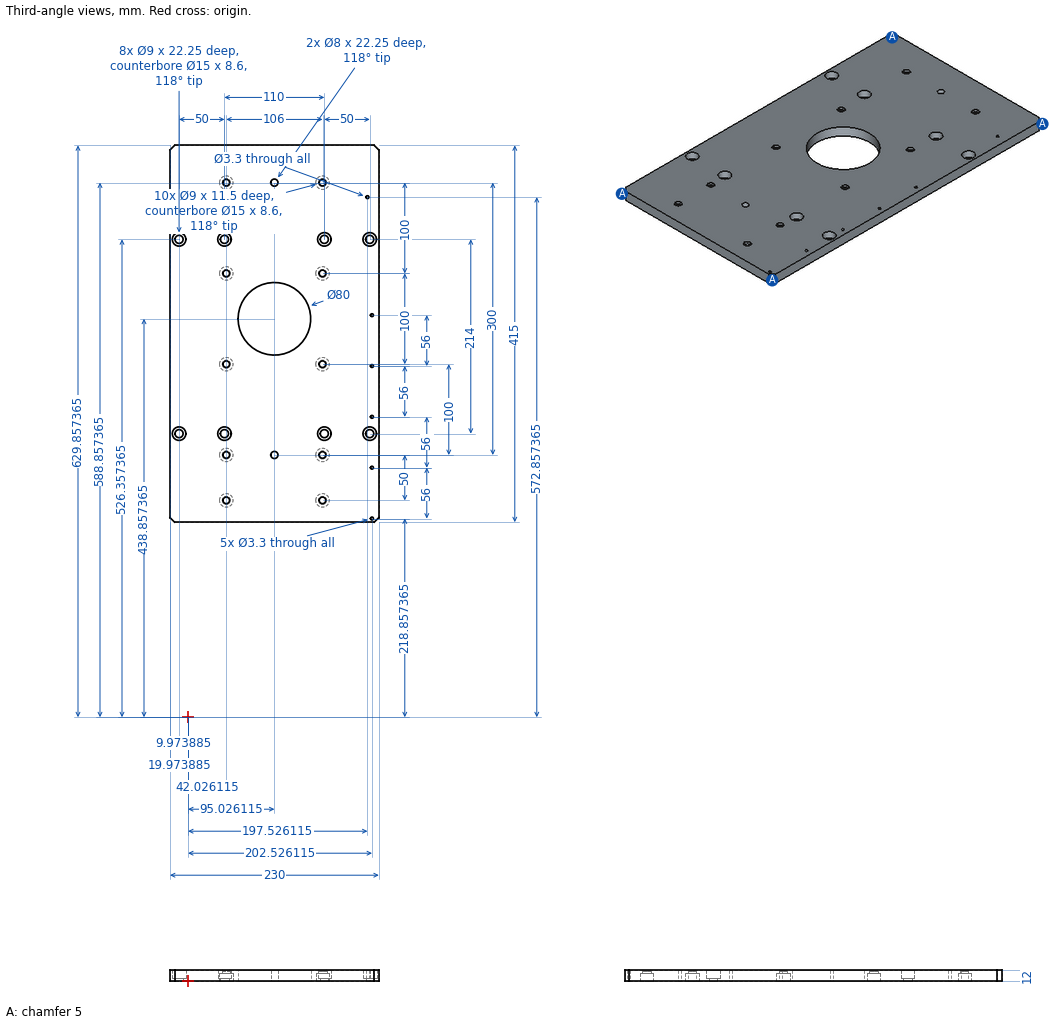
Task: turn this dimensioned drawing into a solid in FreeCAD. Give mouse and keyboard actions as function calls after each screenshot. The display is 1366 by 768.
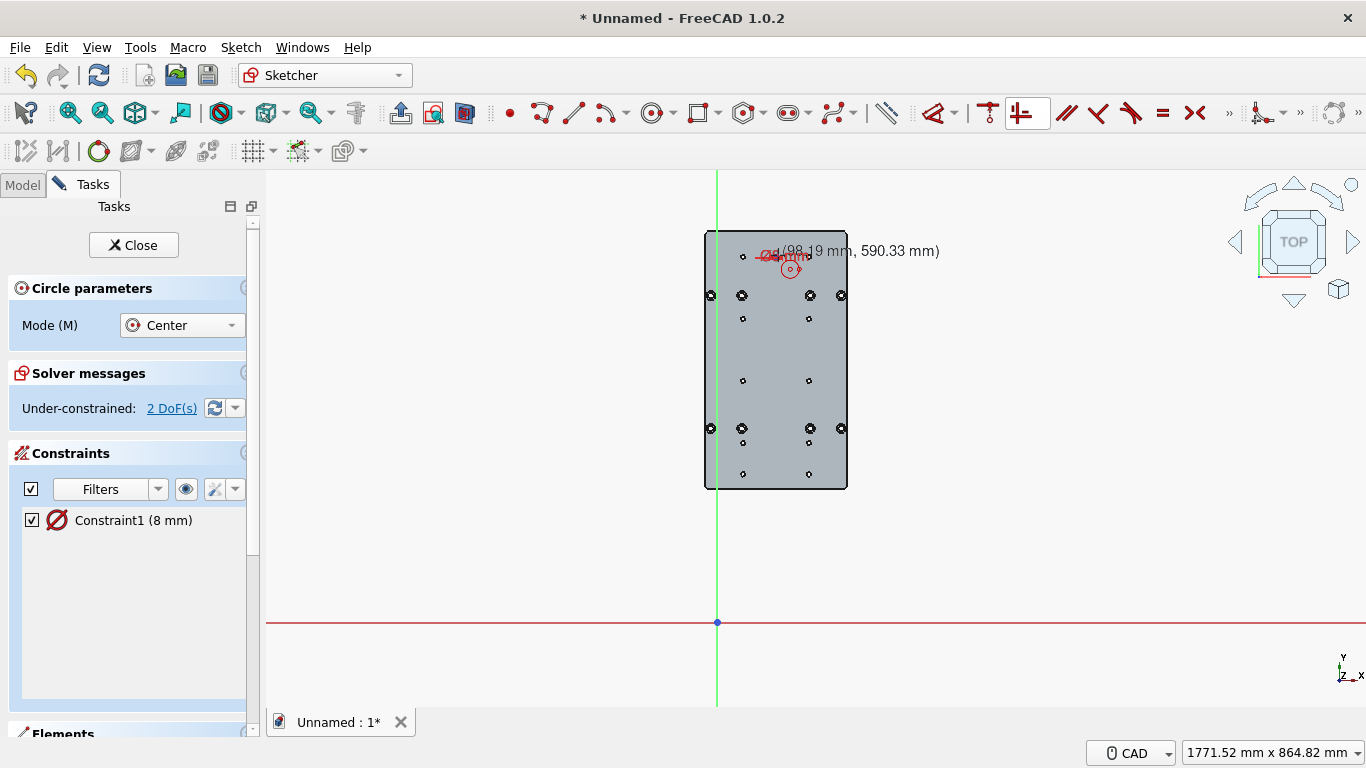
scroll(776, 443, up, 12)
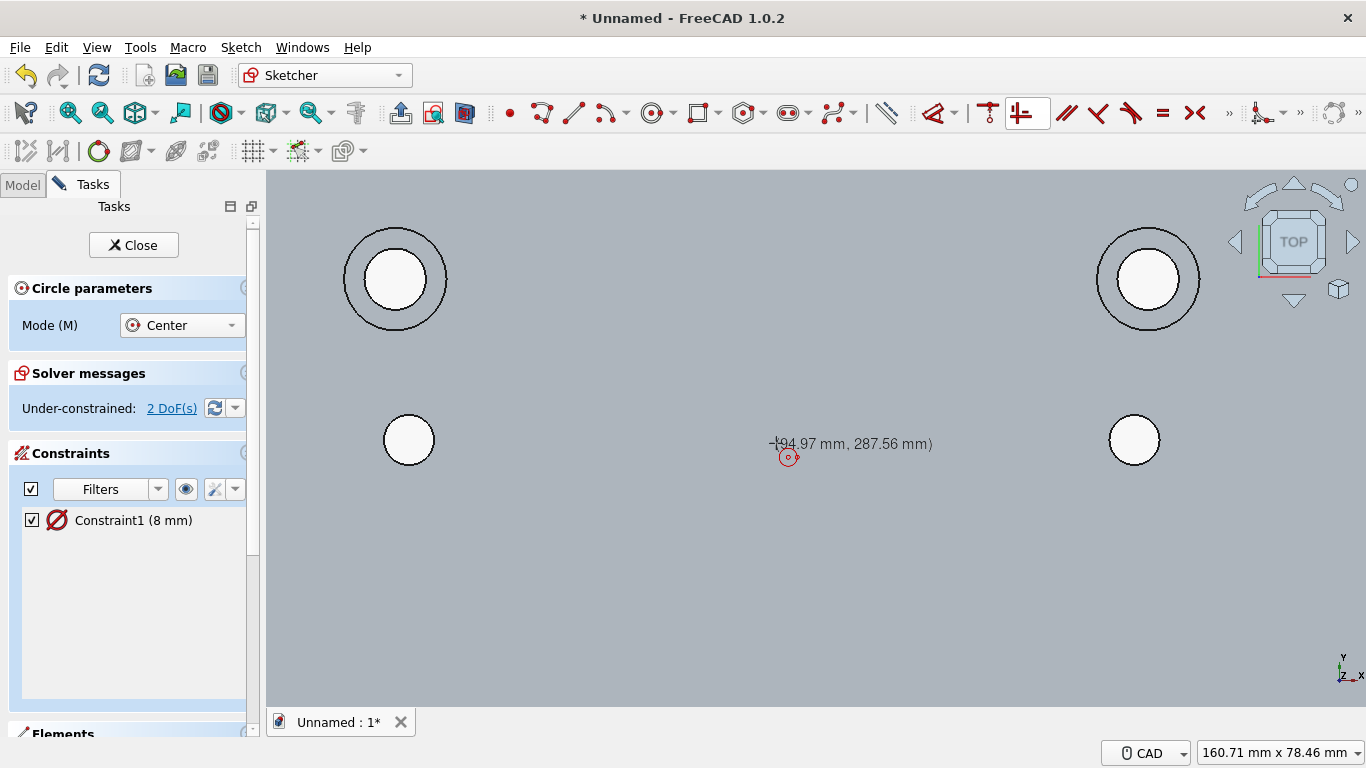
scroll(776, 444, down, 12)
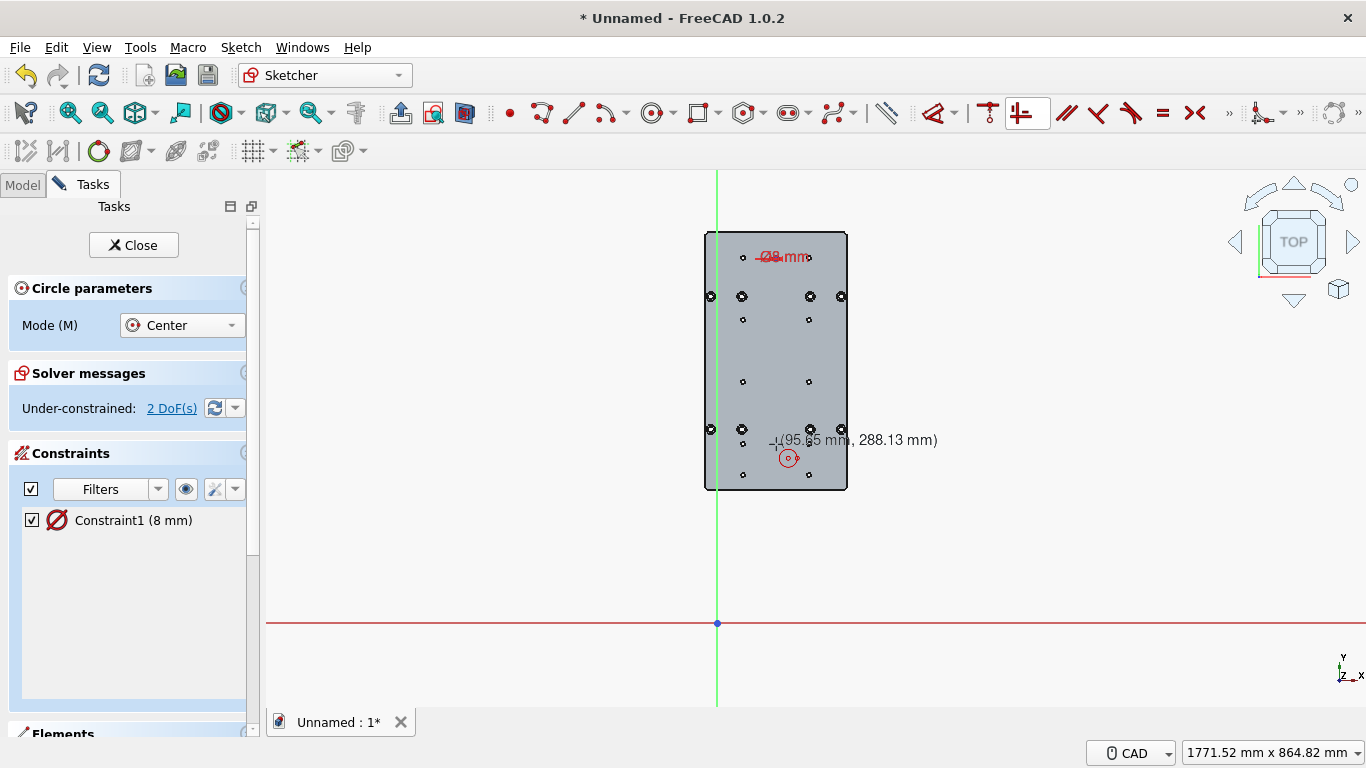
click(776, 444)
move(778, 442)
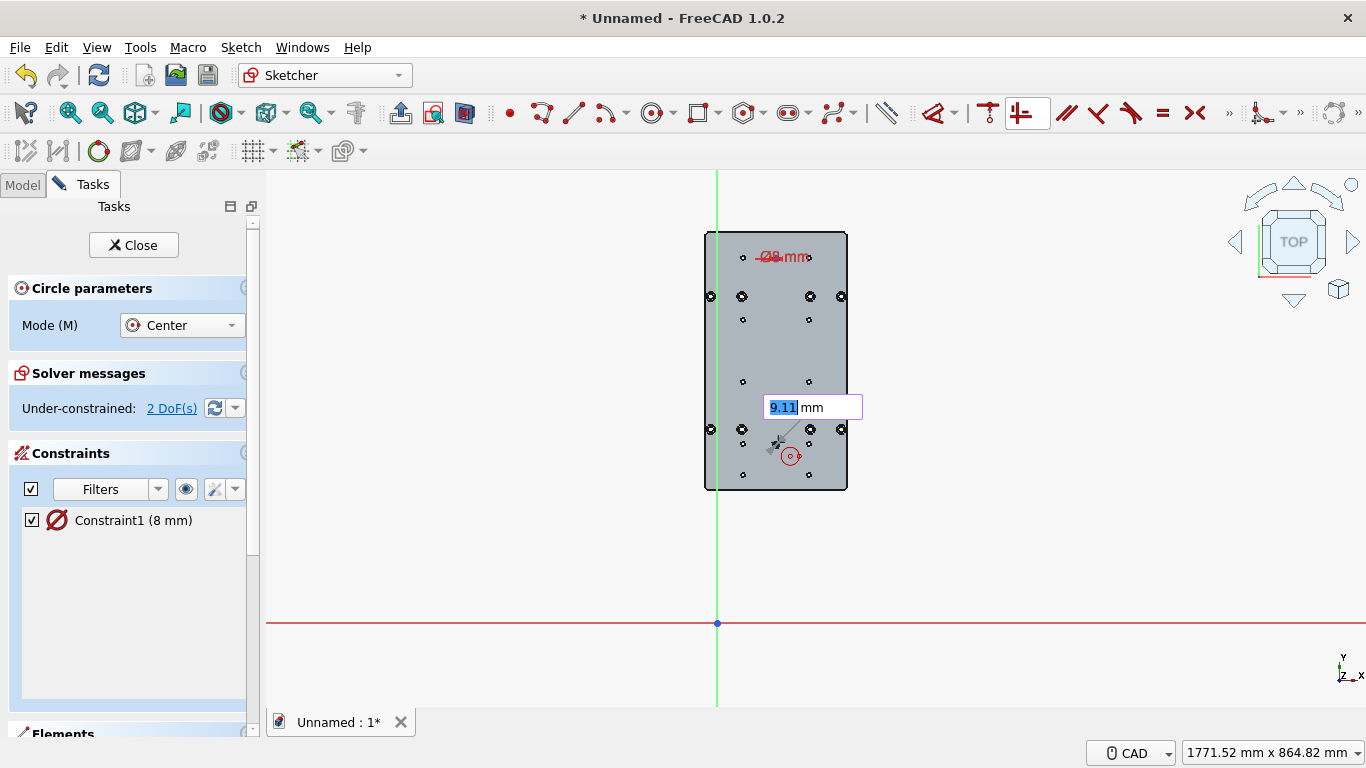
text(8)
key(Return)
key(Escape)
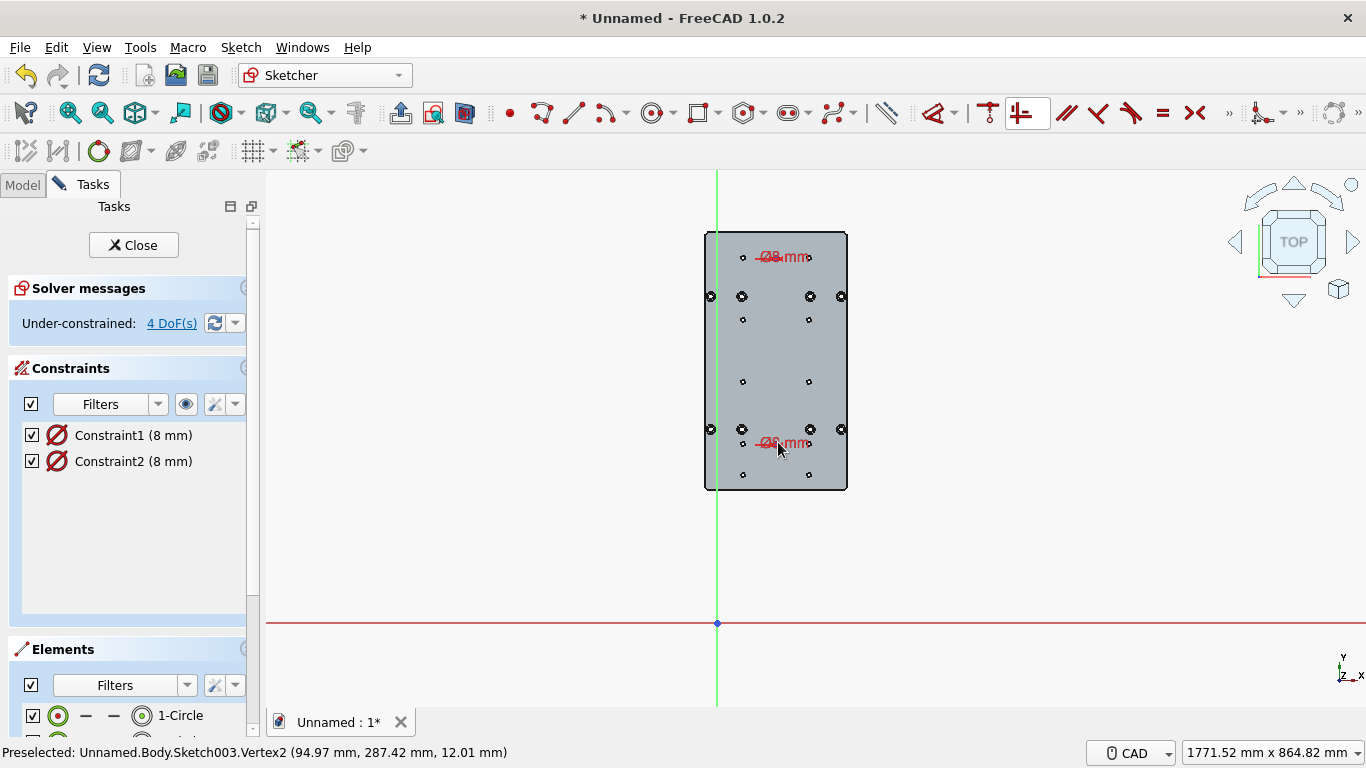
click(776, 259)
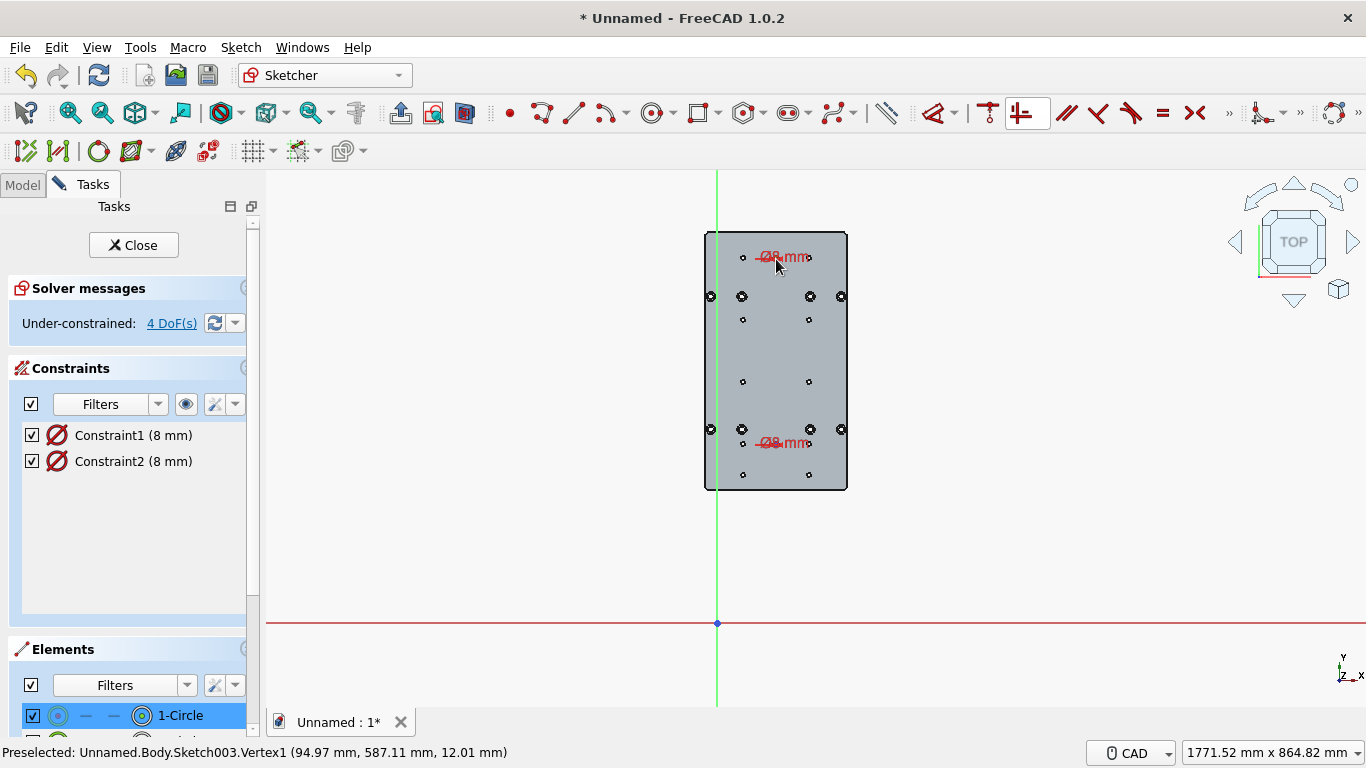
click(776, 445)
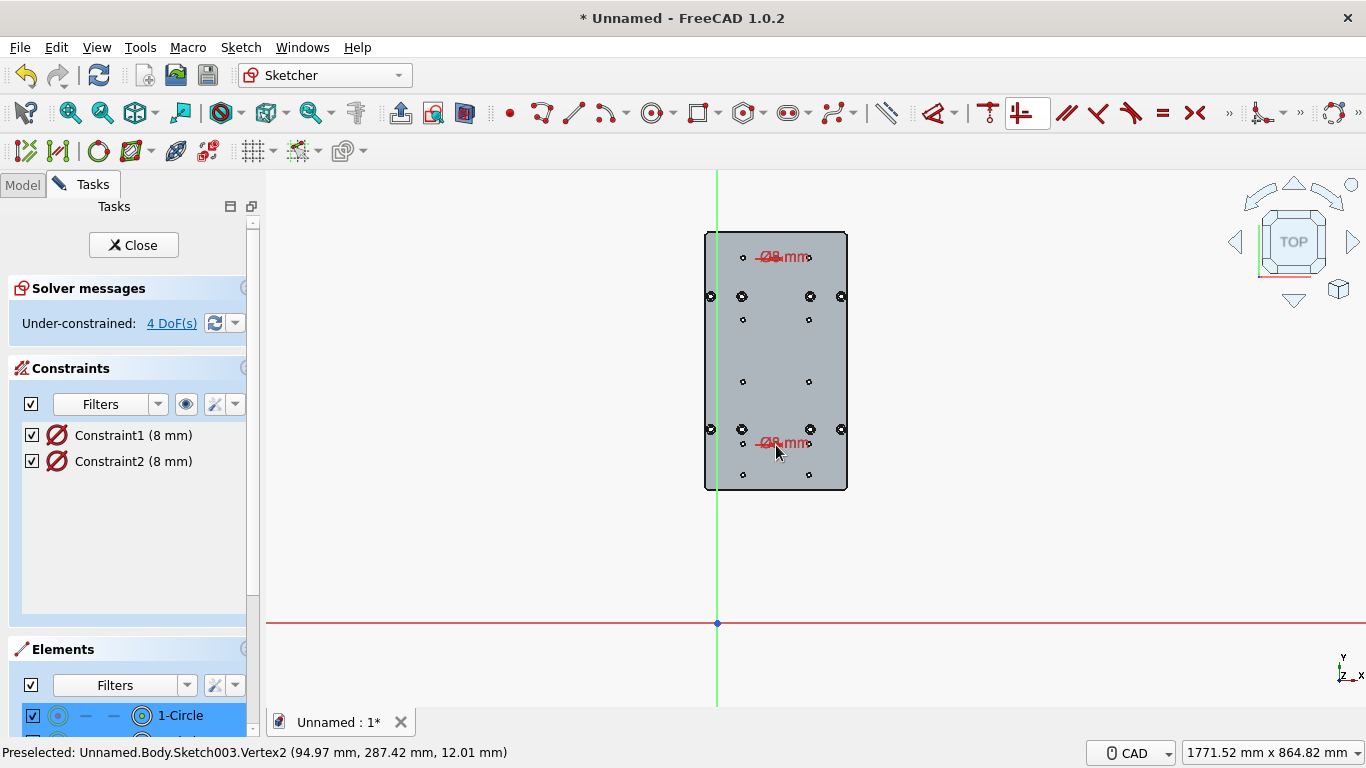
click(1044, 114)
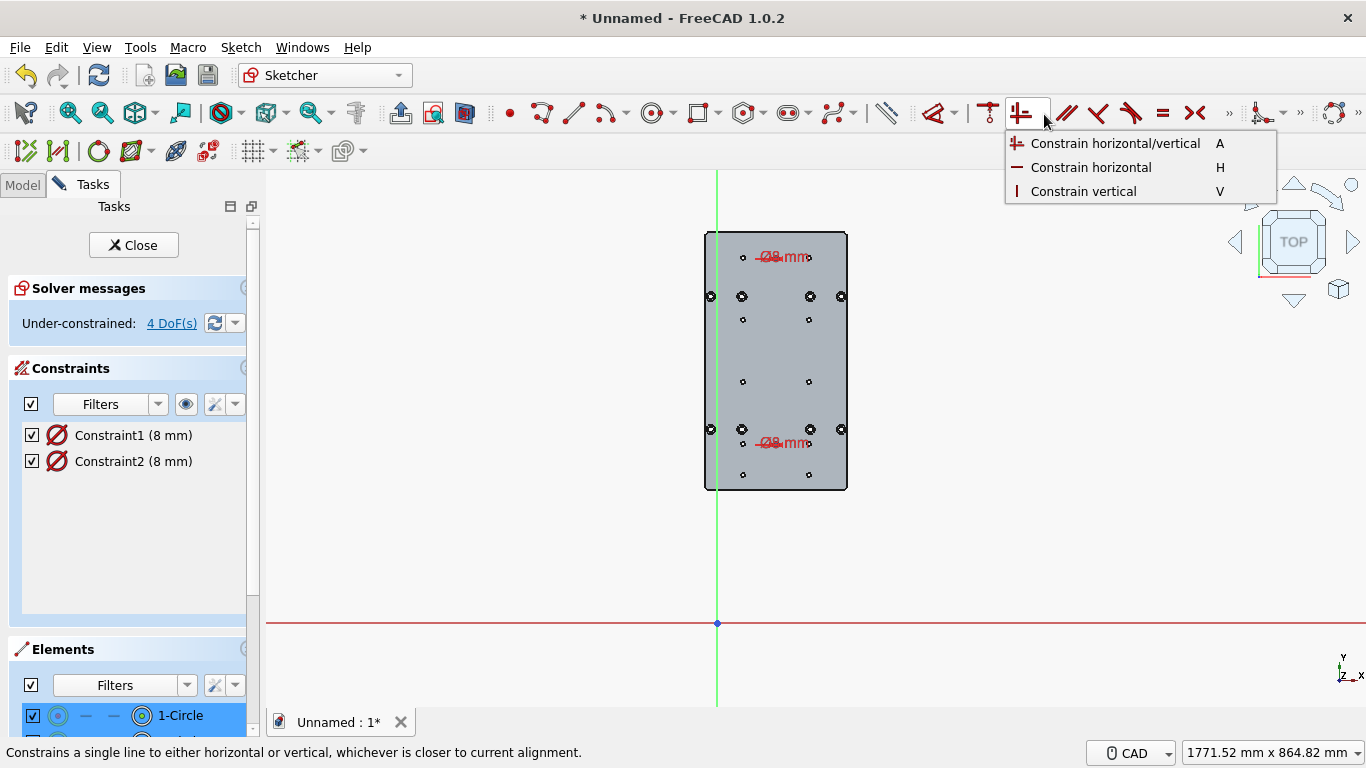
click(1141, 191)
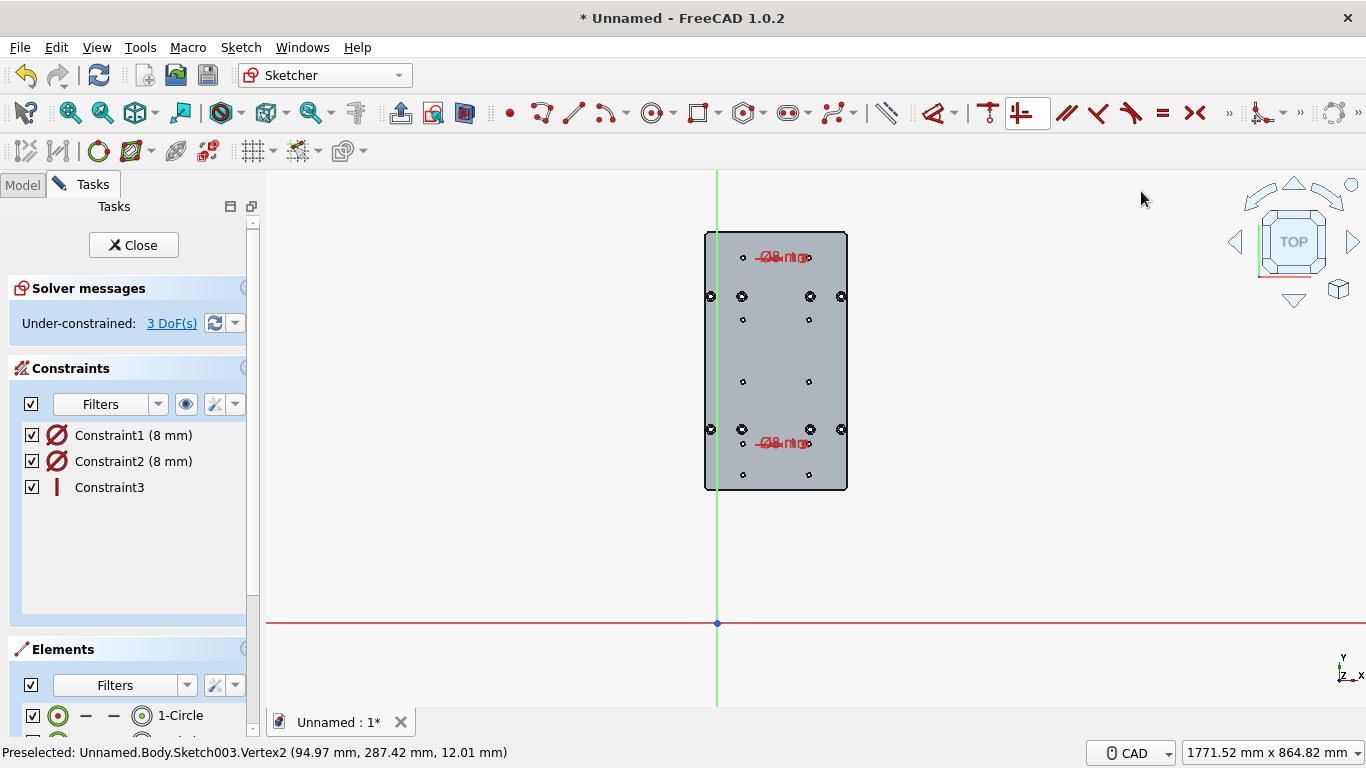
click(934, 114)